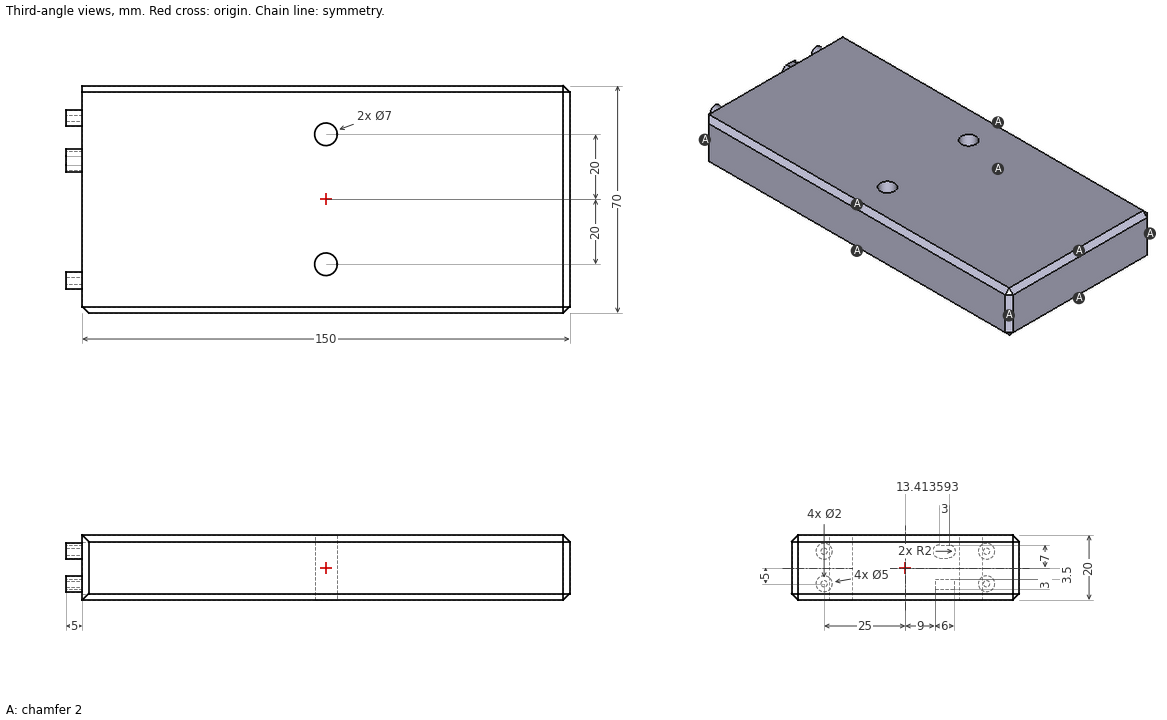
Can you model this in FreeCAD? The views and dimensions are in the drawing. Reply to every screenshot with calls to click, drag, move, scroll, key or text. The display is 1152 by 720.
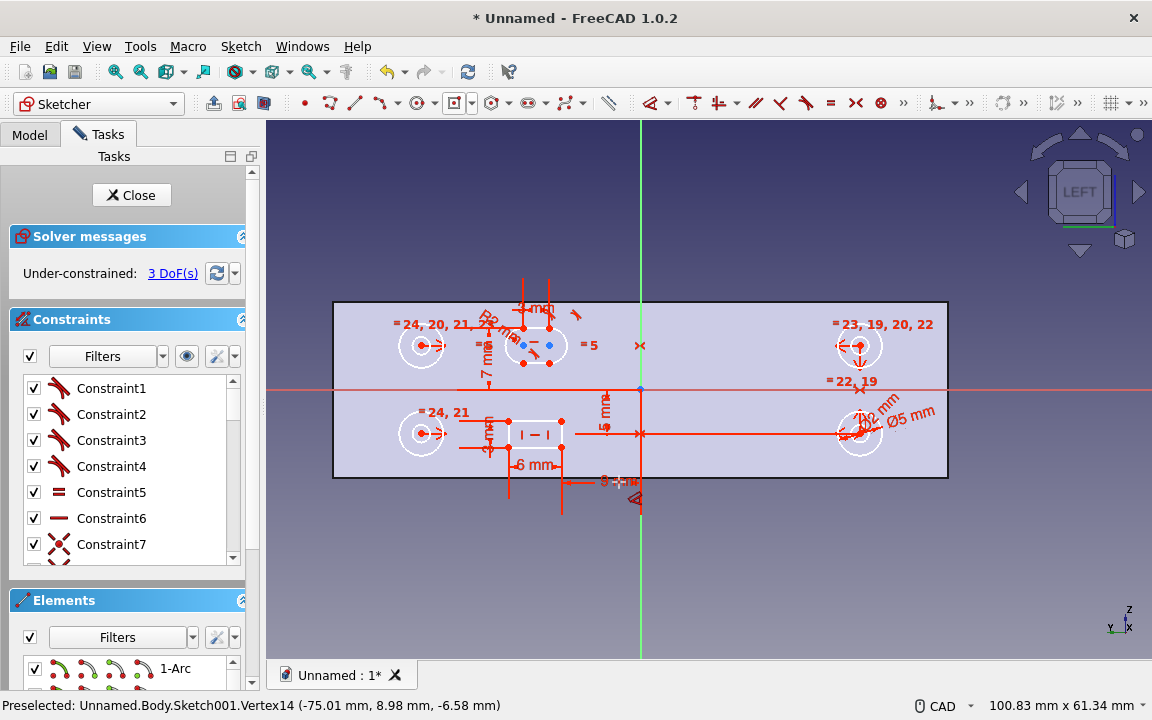
click(860, 434)
click(750, 468)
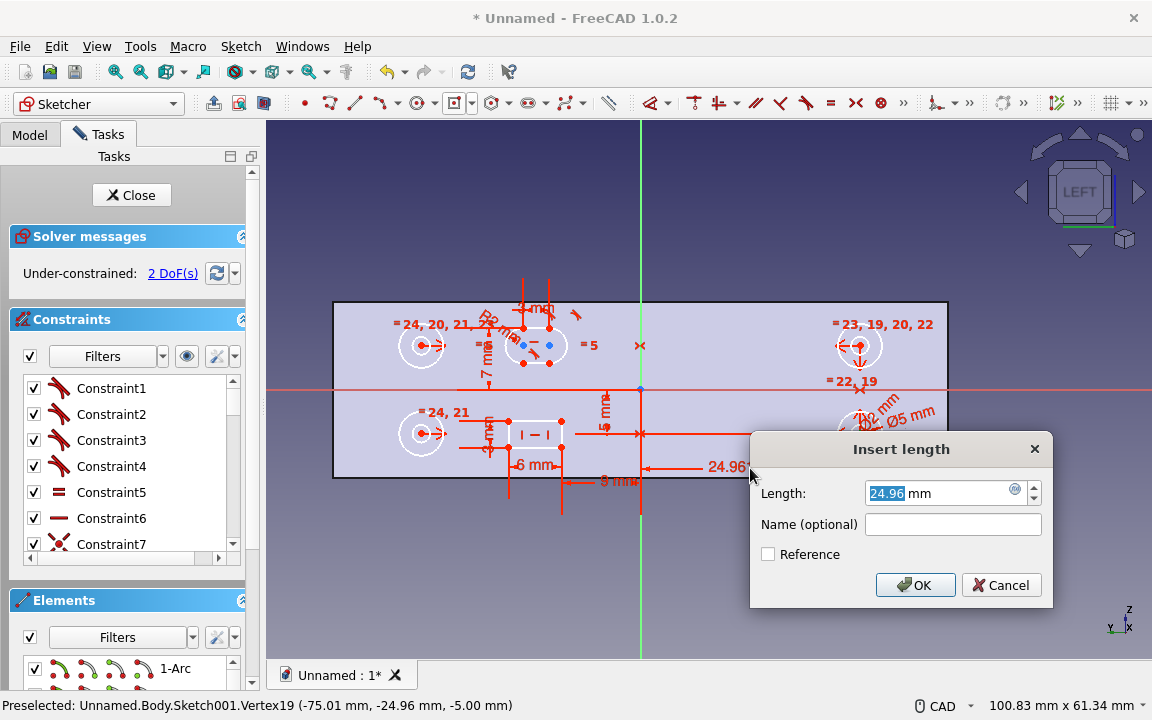
text(25)
key(Return)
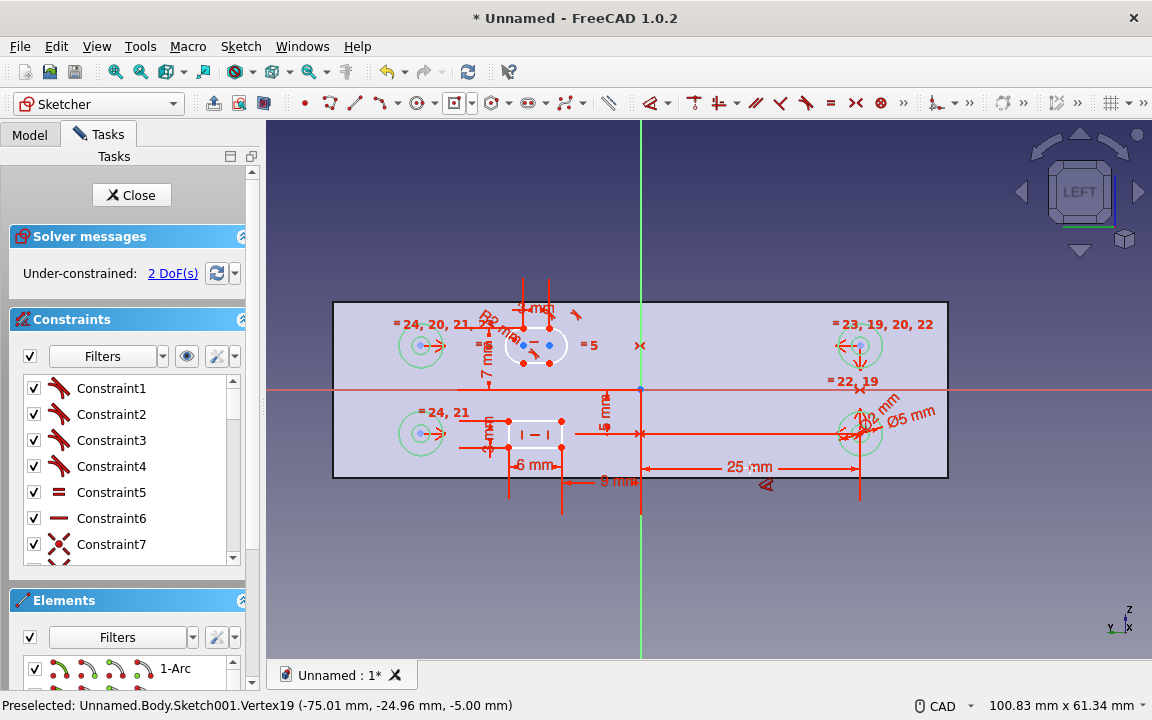
scroll(509, 421, up, 2)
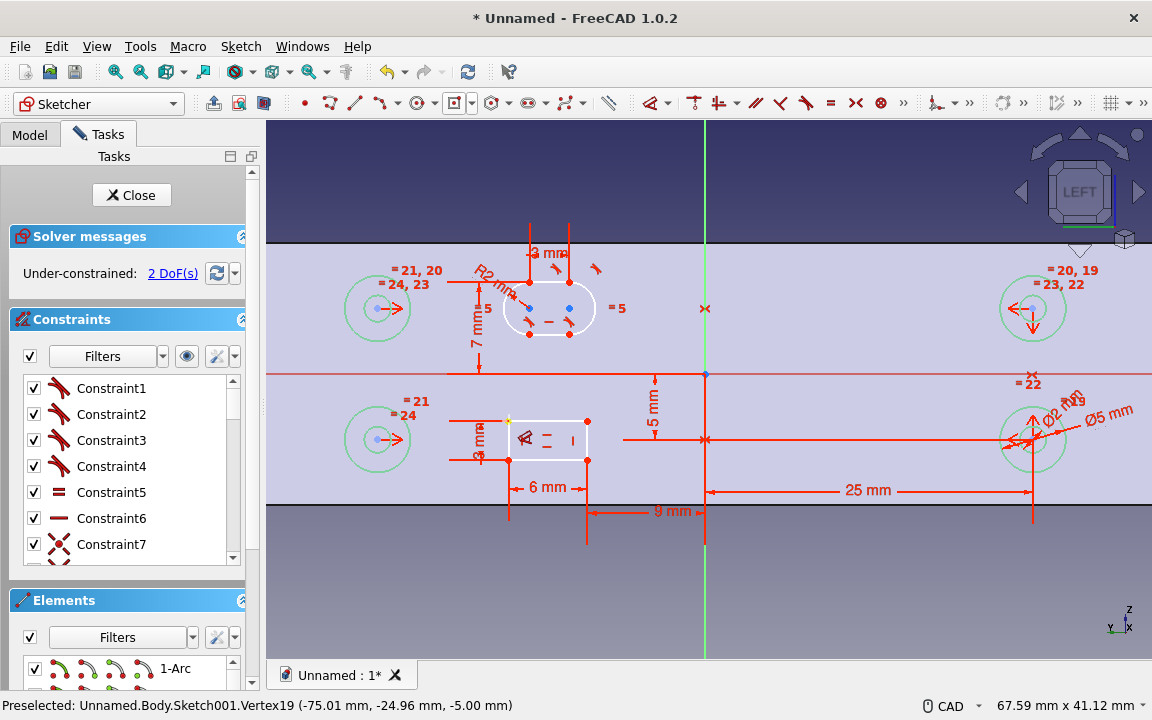
click(509, 421)
click(475, 398)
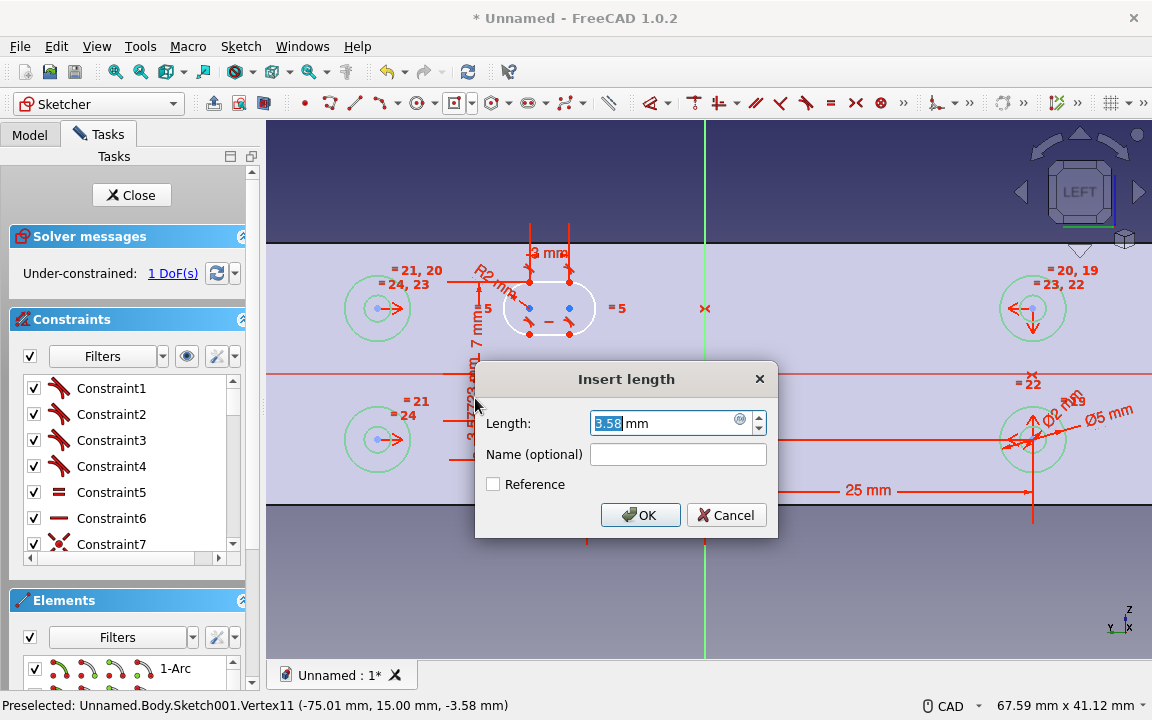
text(3.5)
key(Return)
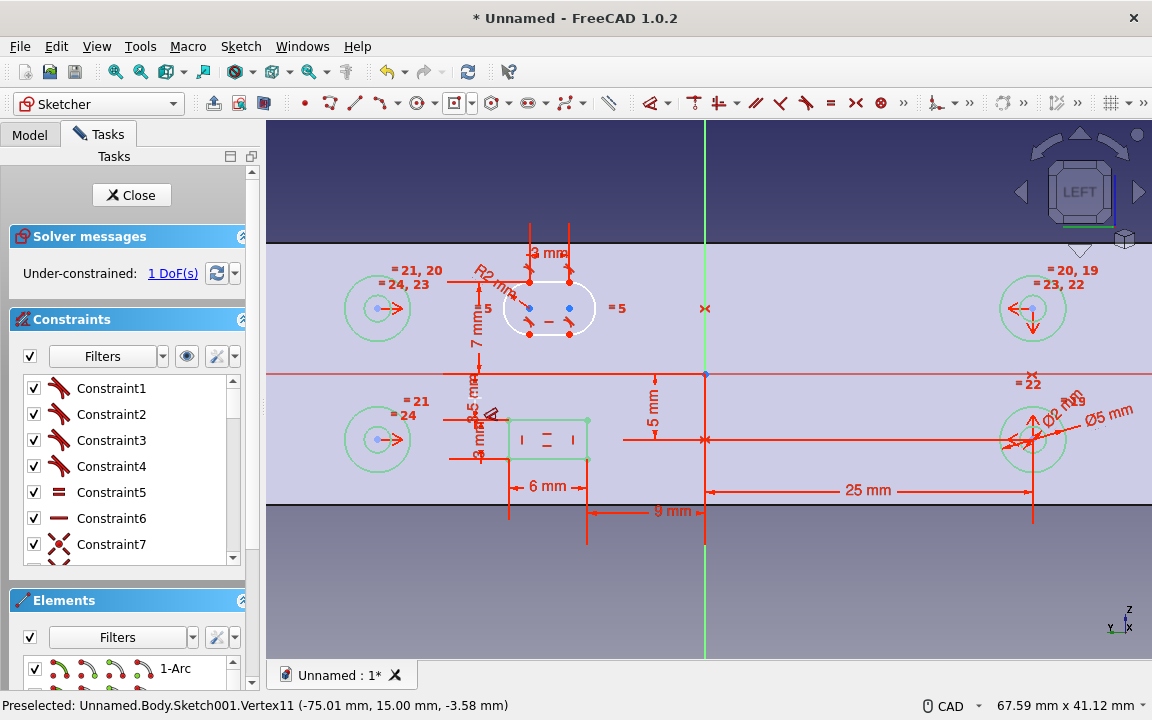
click(530, 282)
click(658, 248)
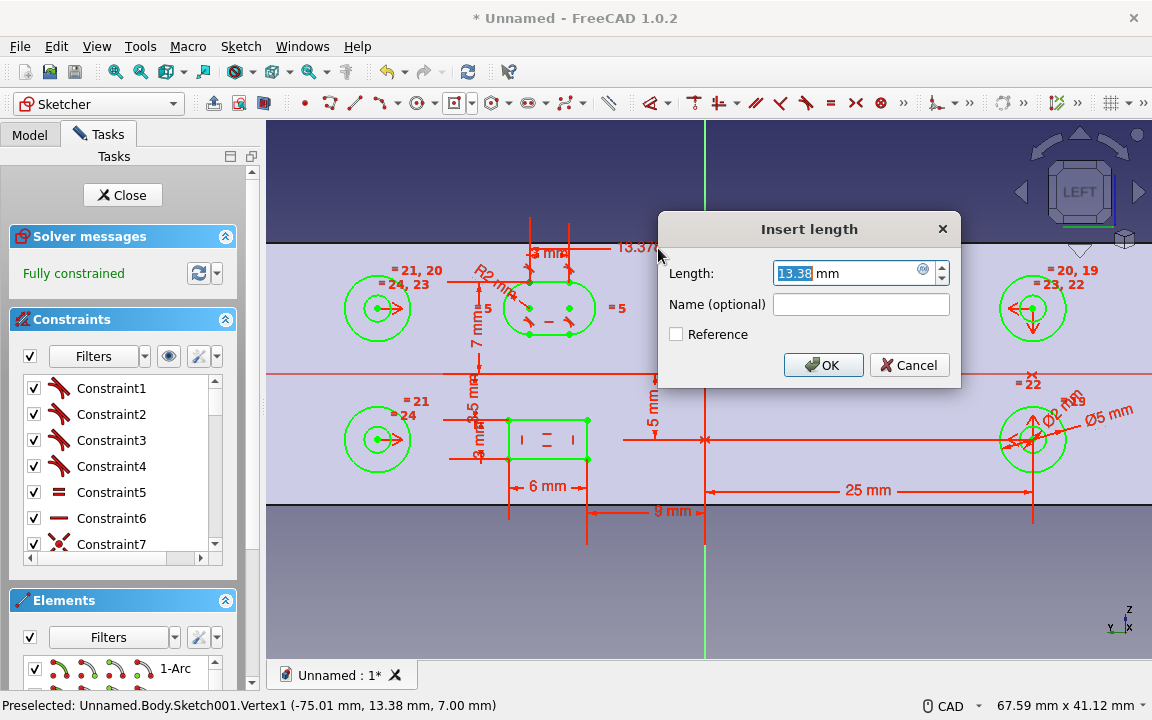
text(13.413593)
key(Return)
key(Escape)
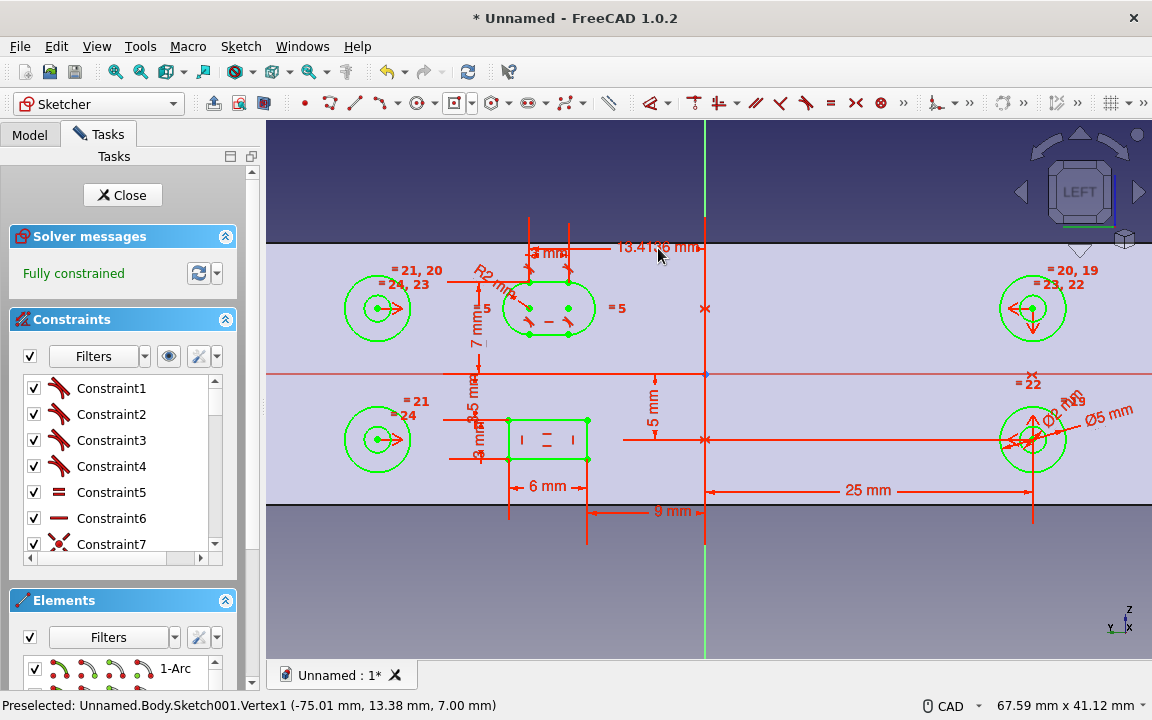
click(123, 195)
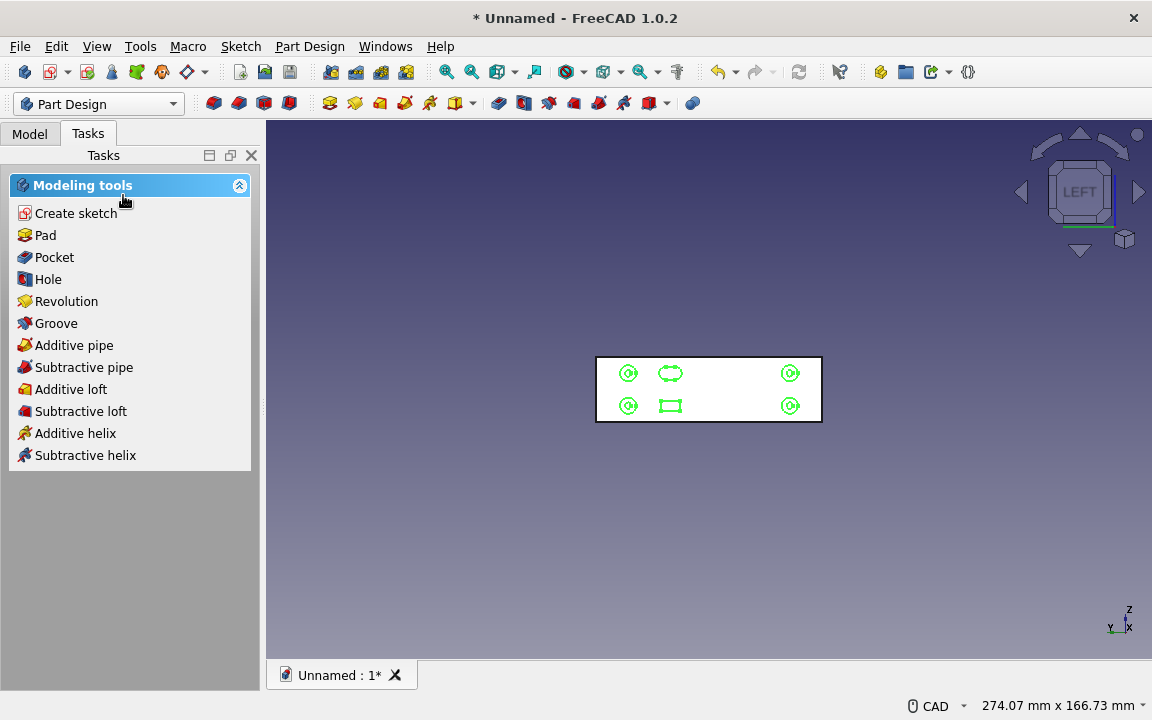
click(330, 104)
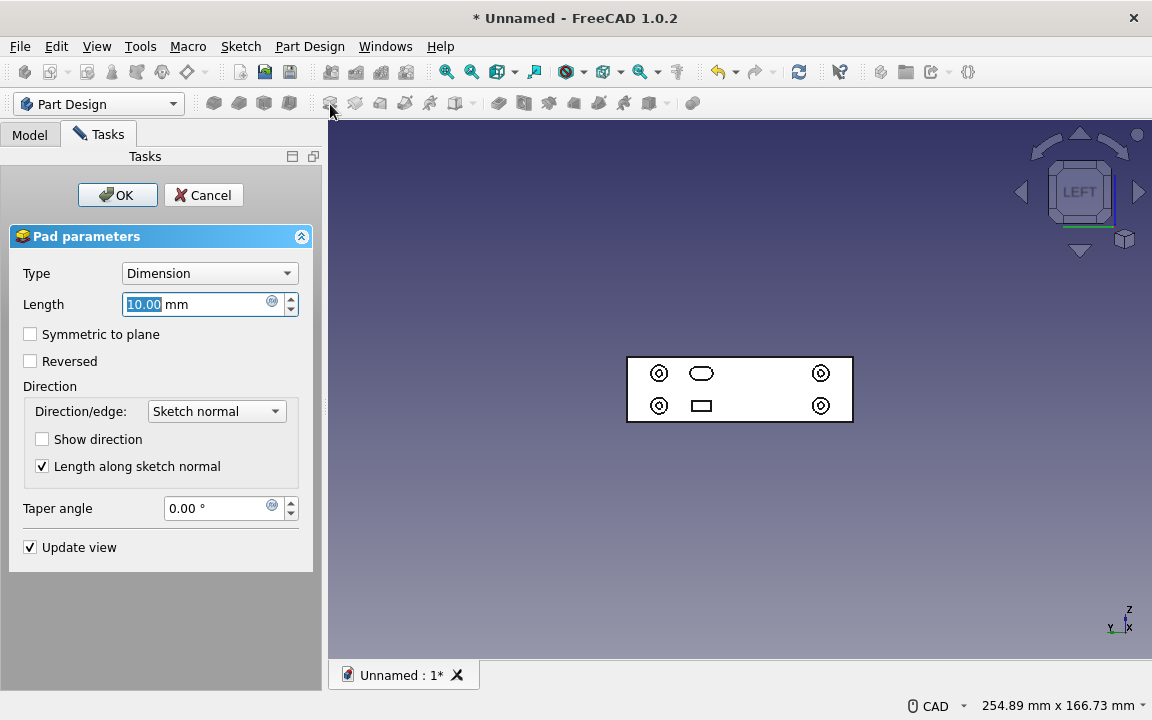
text(5)
key(Tab)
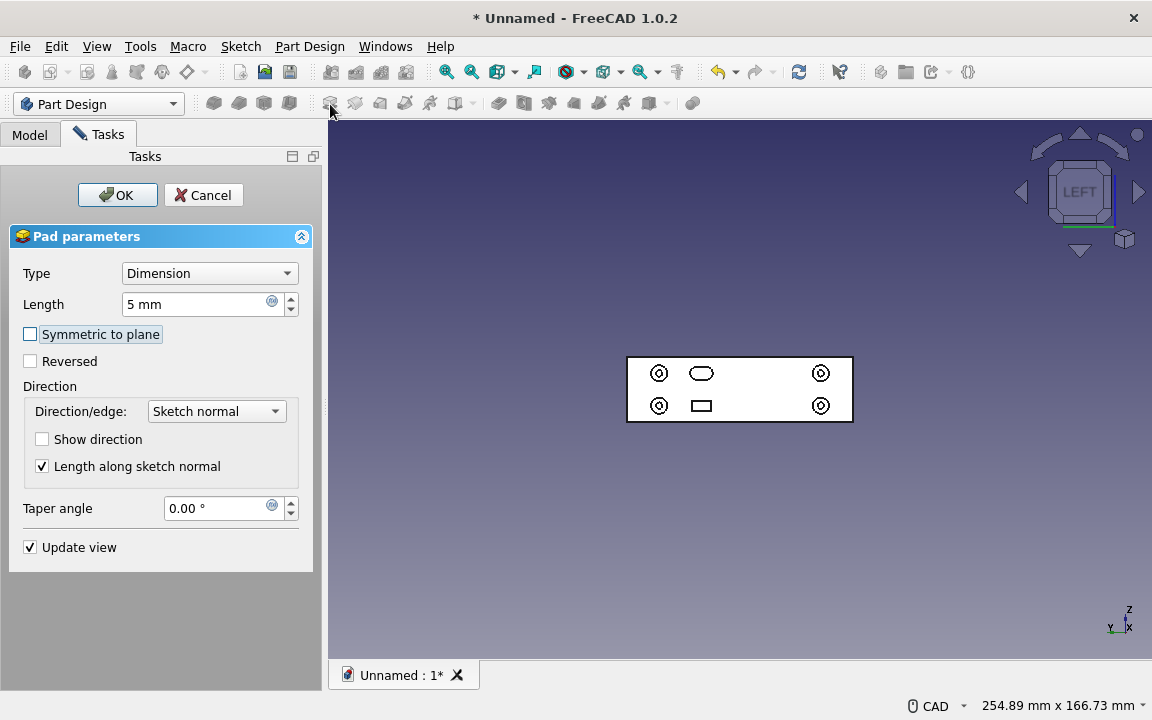
click(118, 195)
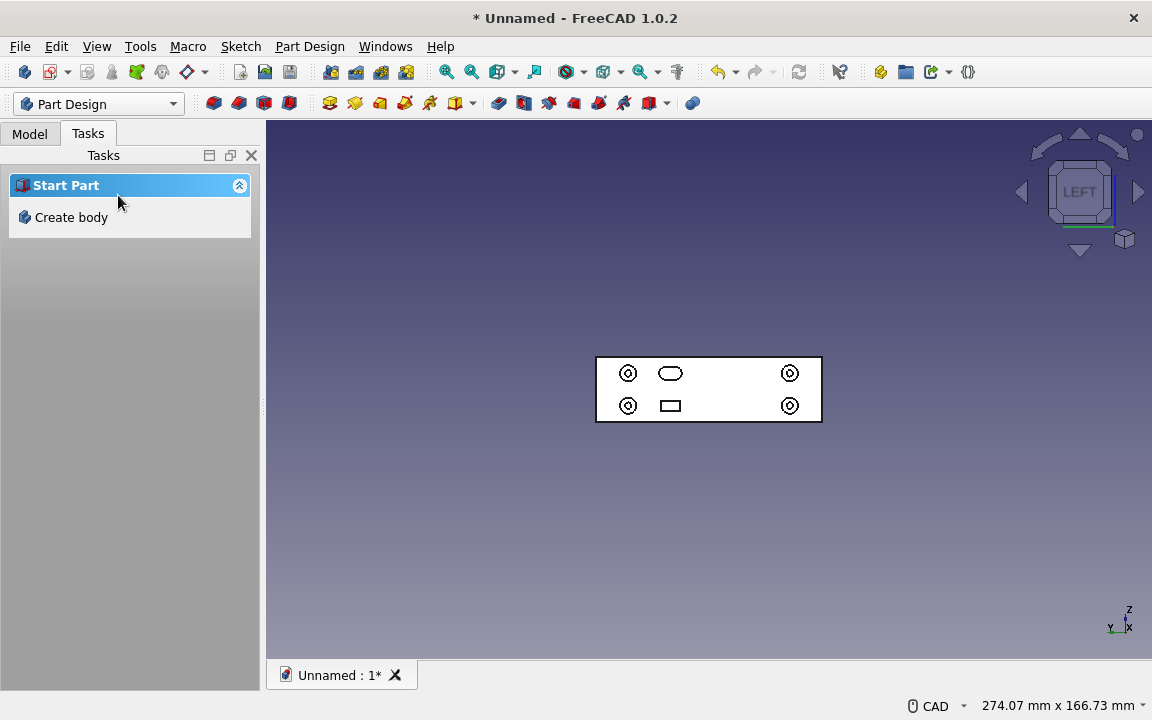
click(447, 72)